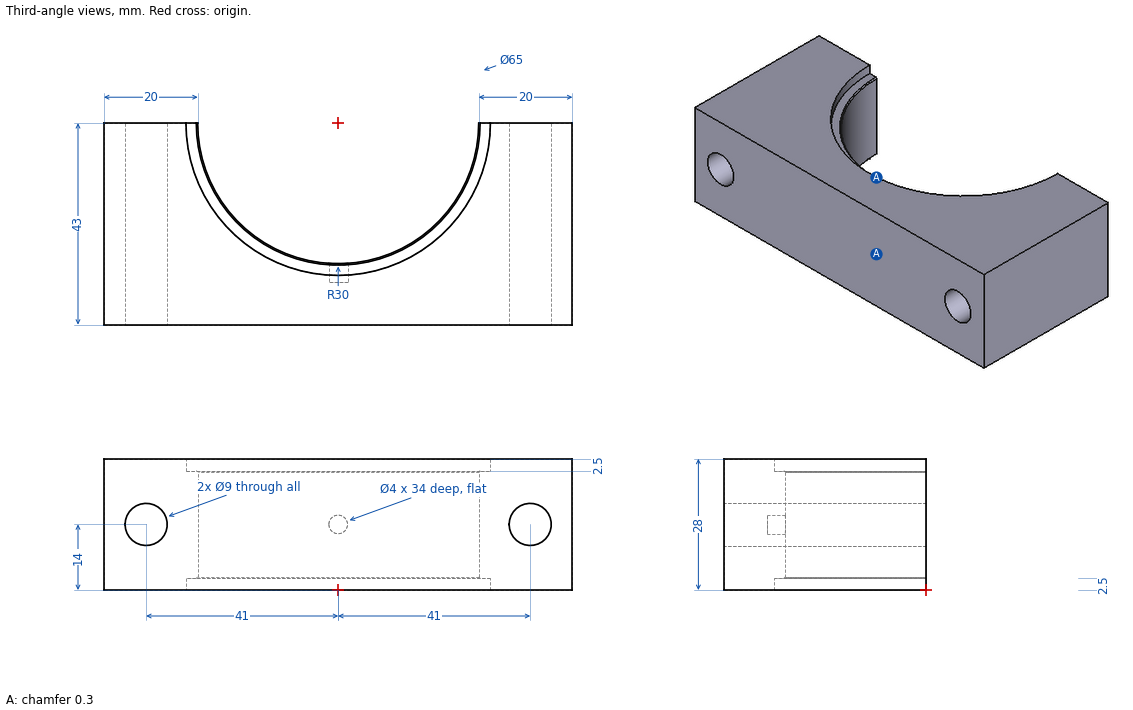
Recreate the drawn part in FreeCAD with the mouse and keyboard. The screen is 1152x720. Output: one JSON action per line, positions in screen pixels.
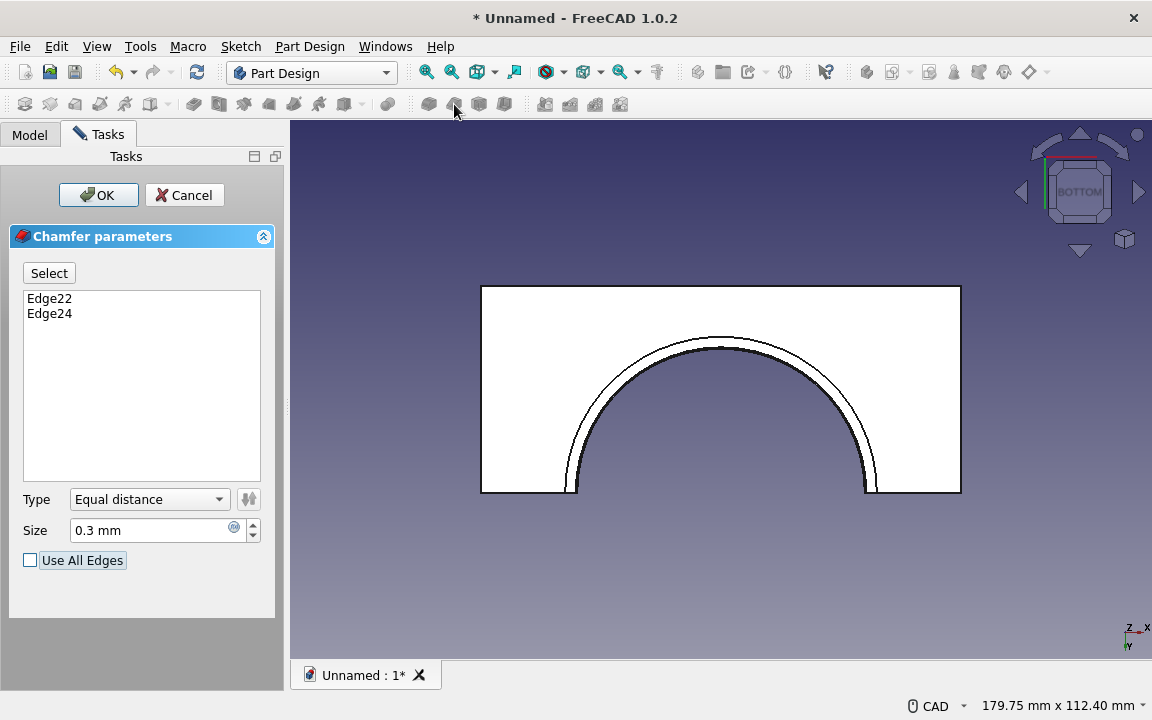
{"action": "left_click", "coordinate": [99, 195]}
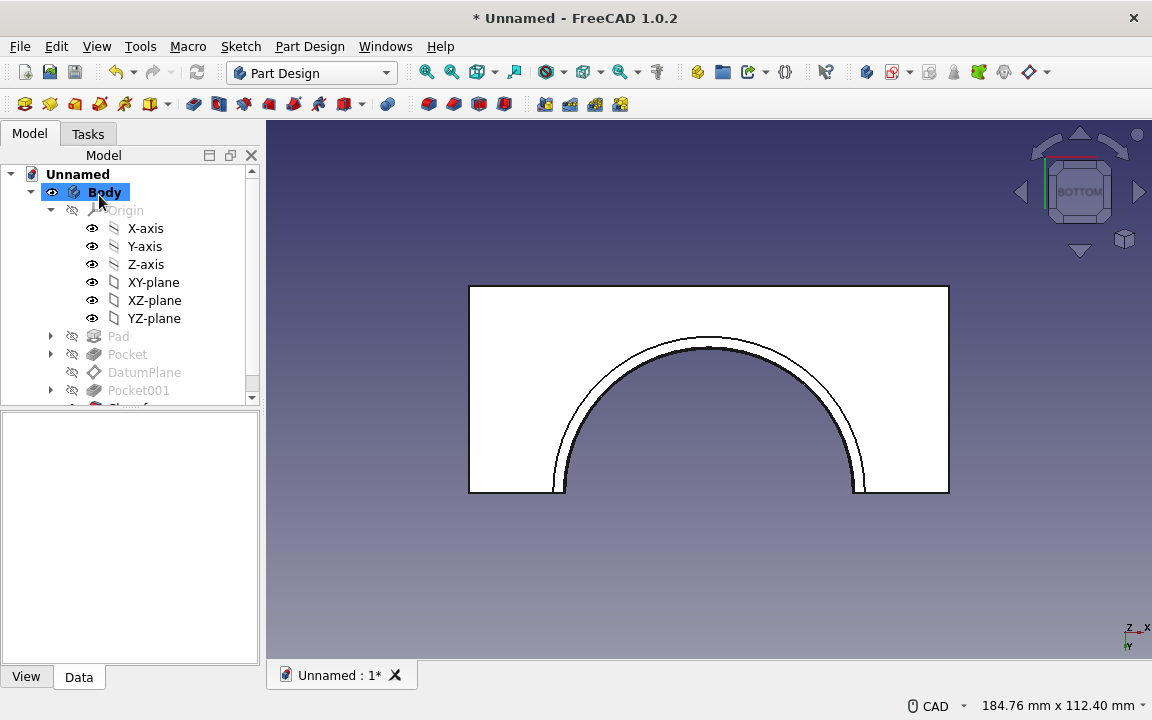
{"action": "left_click", "coordinate": [892, 72]}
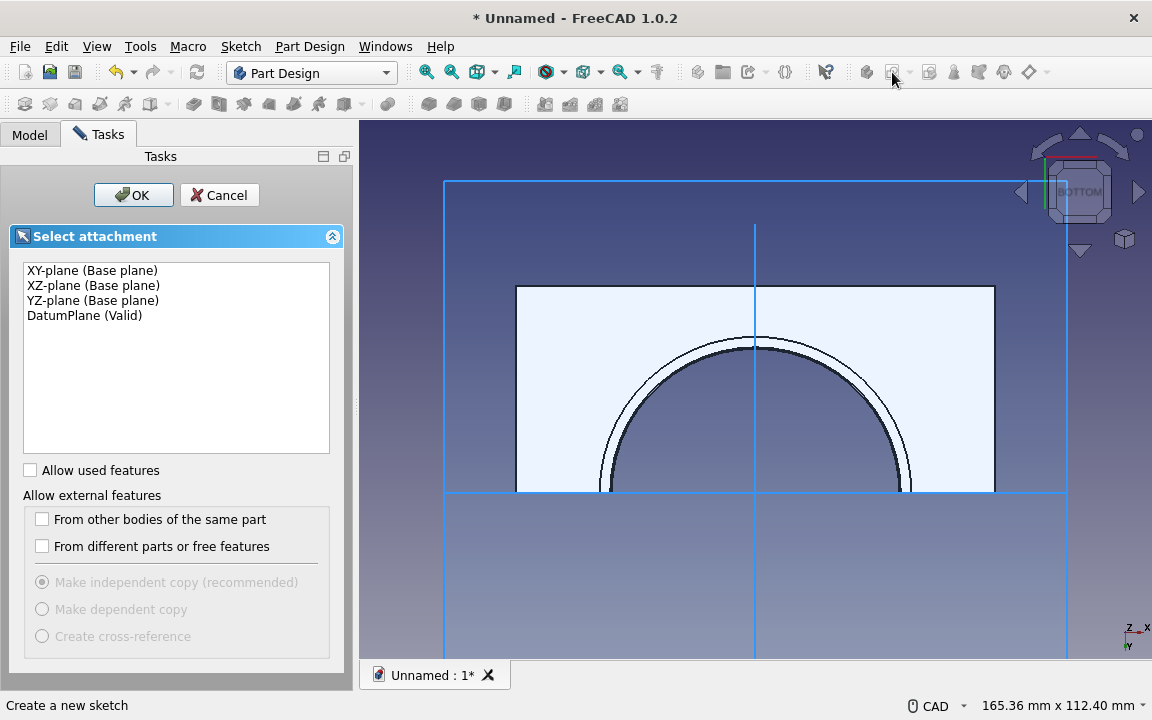
{"action": "left_click", "coordinate": [84, 286]}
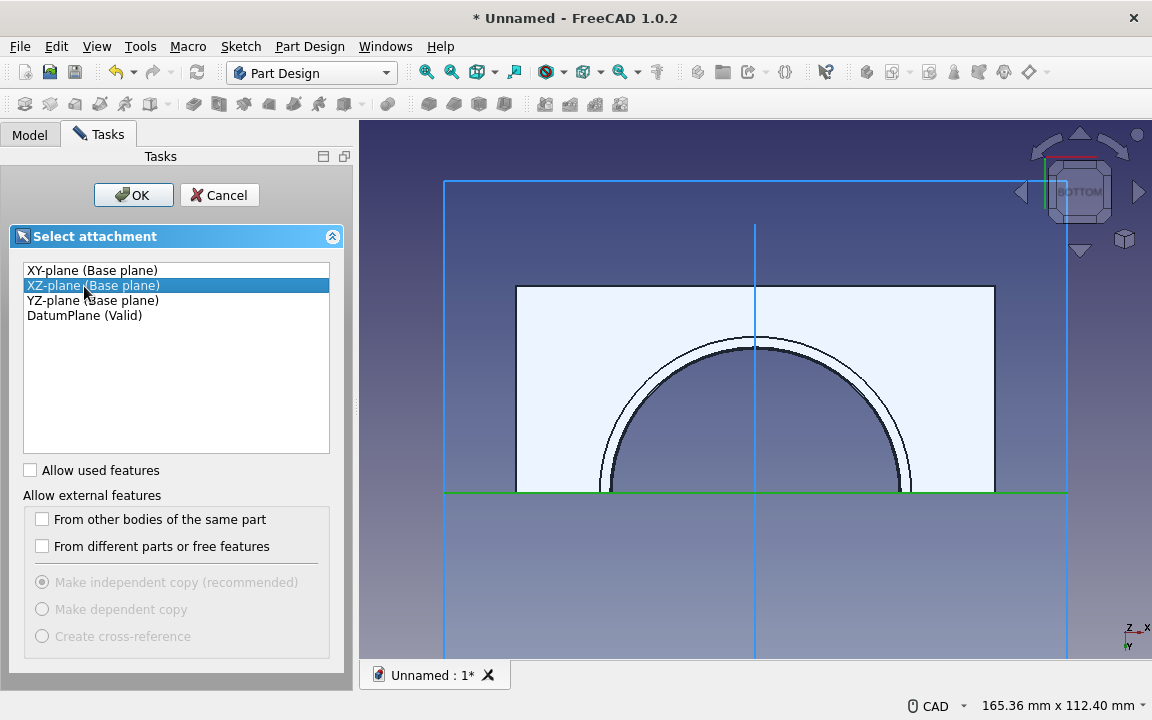
{"action": "left_click", "coordinate": [134, 195]}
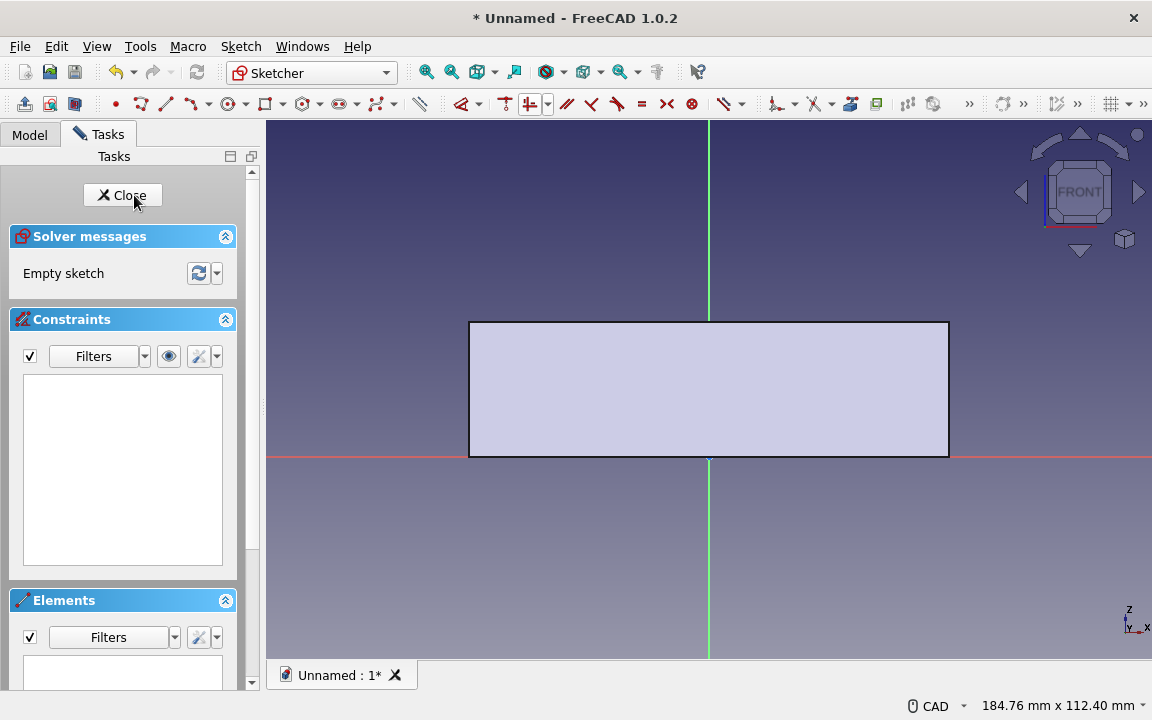
{"action": "left_click", "coordinate": [75, 104]}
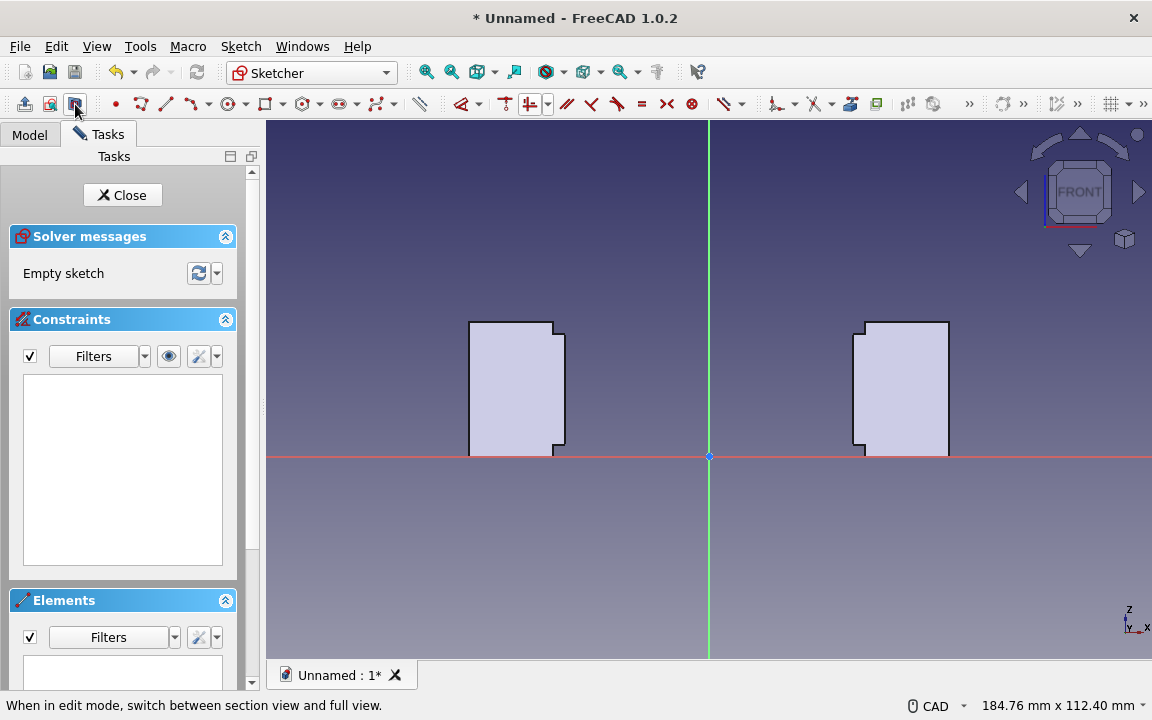
{"action": "left_click", "coordinate": [228, 104]}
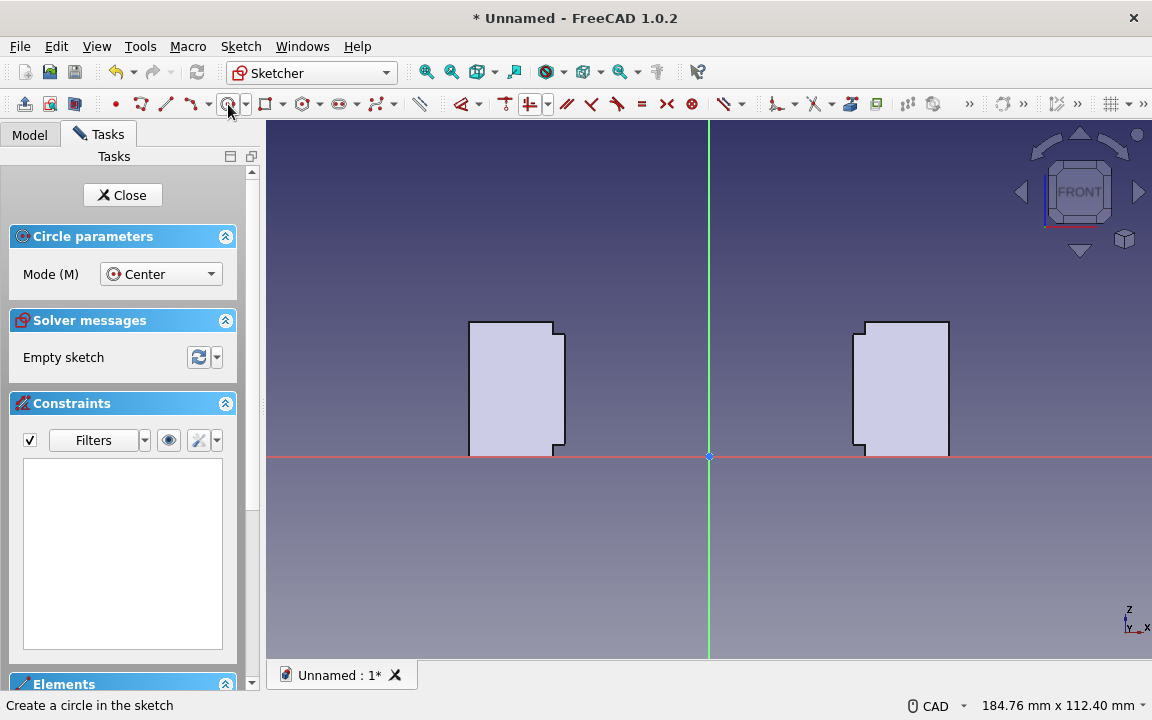
{"action": "left_click", "coordinate": [512, 390]}
{"action": "left_click", "coordinate": [528, 374]}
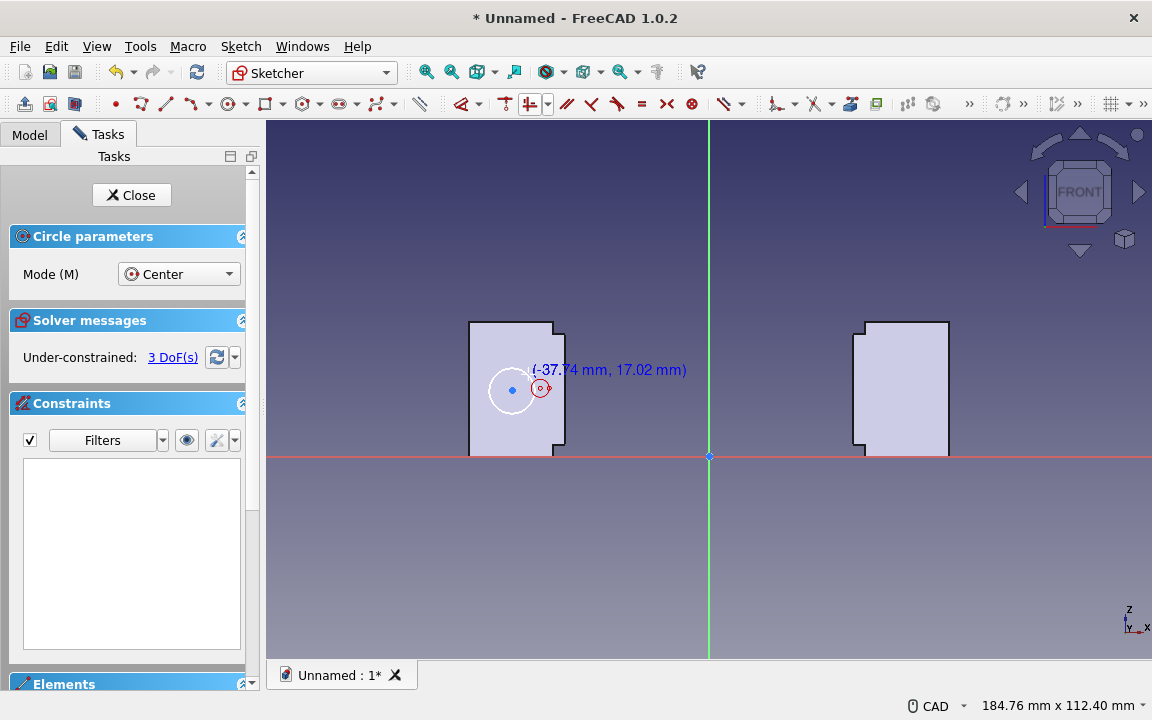
{"action": "left_click", "coordinate": [906, 390]}
{"action": "left_click", "coordinate": [921, 374]}
{"action": "key", "text": "Escape"}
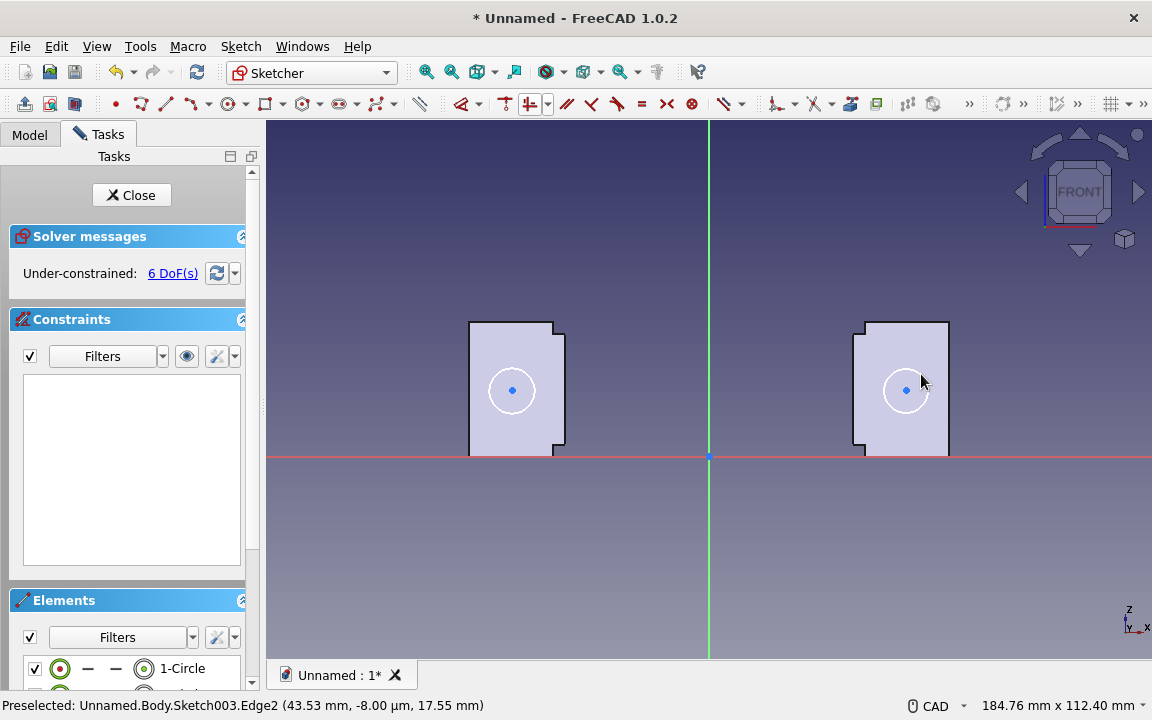
{"action": "left_click", "coordinate": [528, 375]}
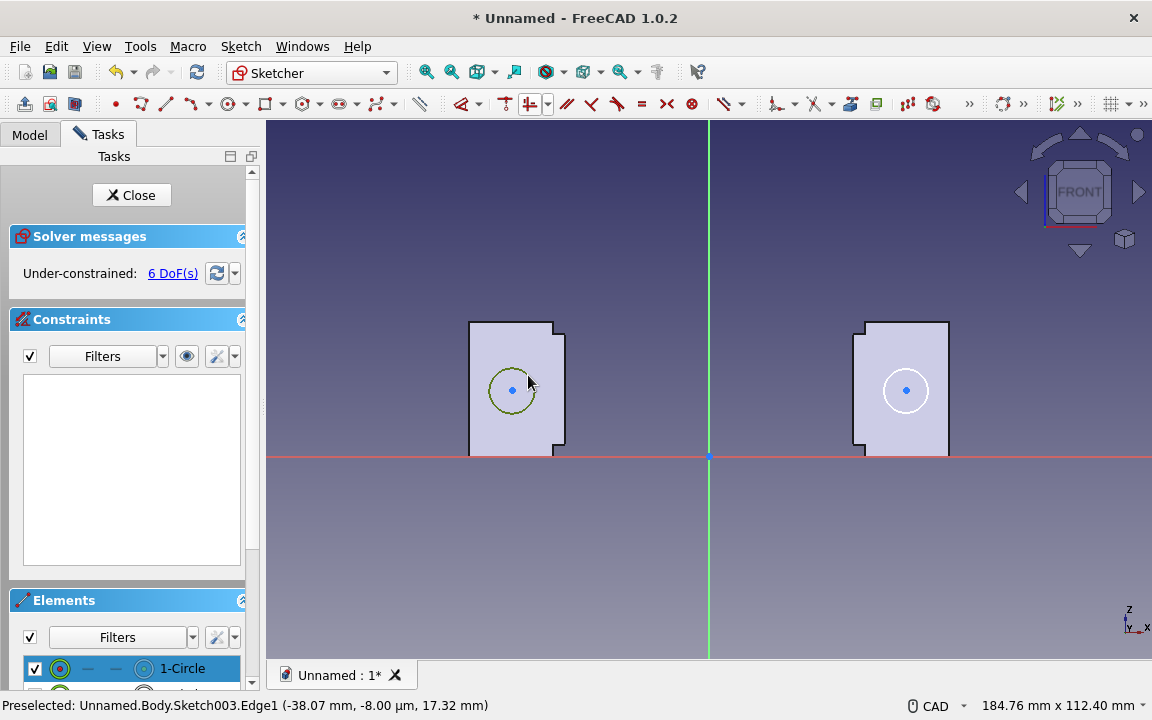
{"action": "left_click", "coordinate": [921, 375]}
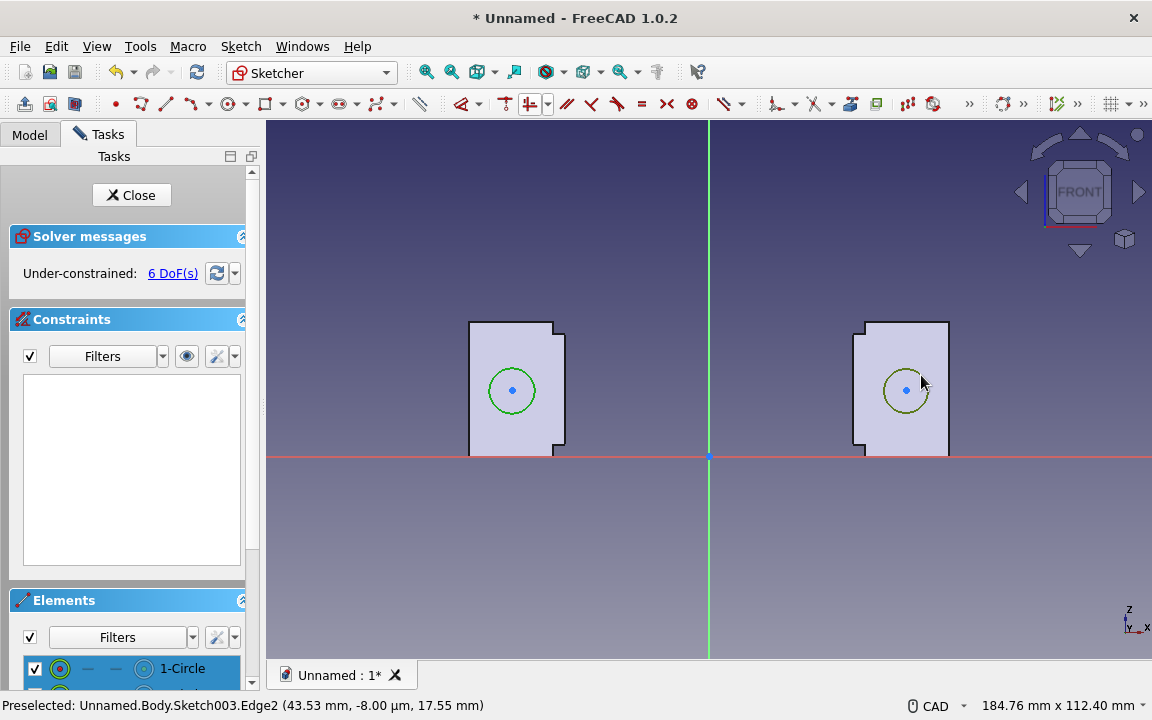
{"action": "left_click", "coordinate": [642, 104]}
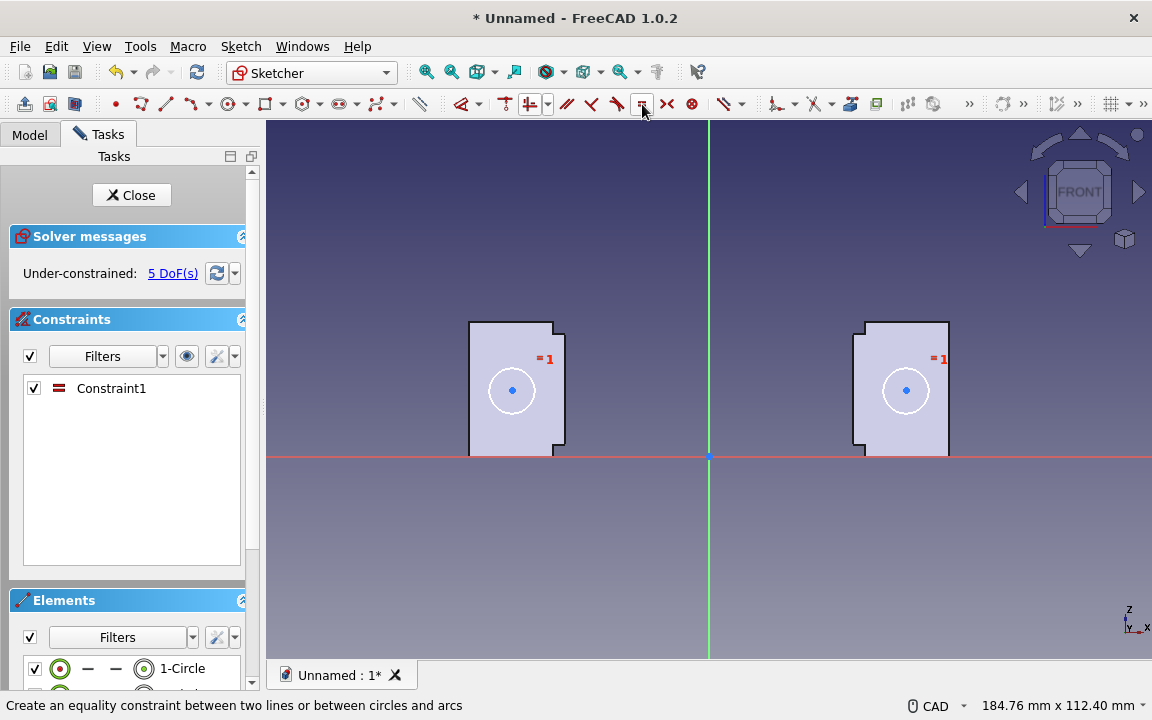
{"action": "left_click", "coordinate": [512, 391]}